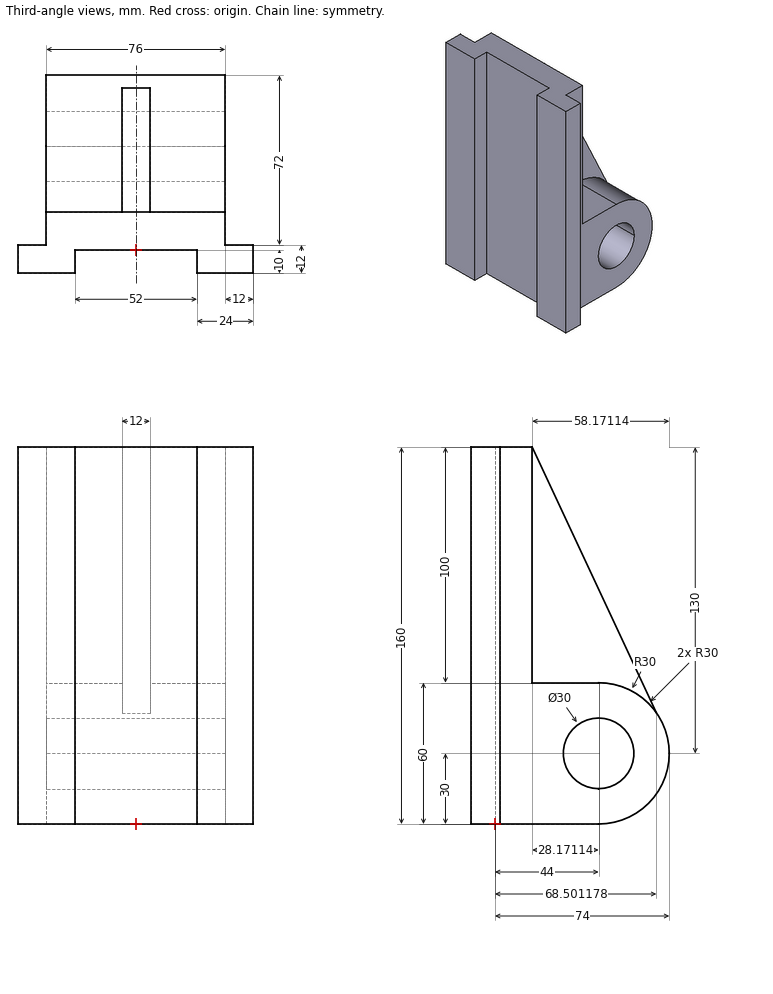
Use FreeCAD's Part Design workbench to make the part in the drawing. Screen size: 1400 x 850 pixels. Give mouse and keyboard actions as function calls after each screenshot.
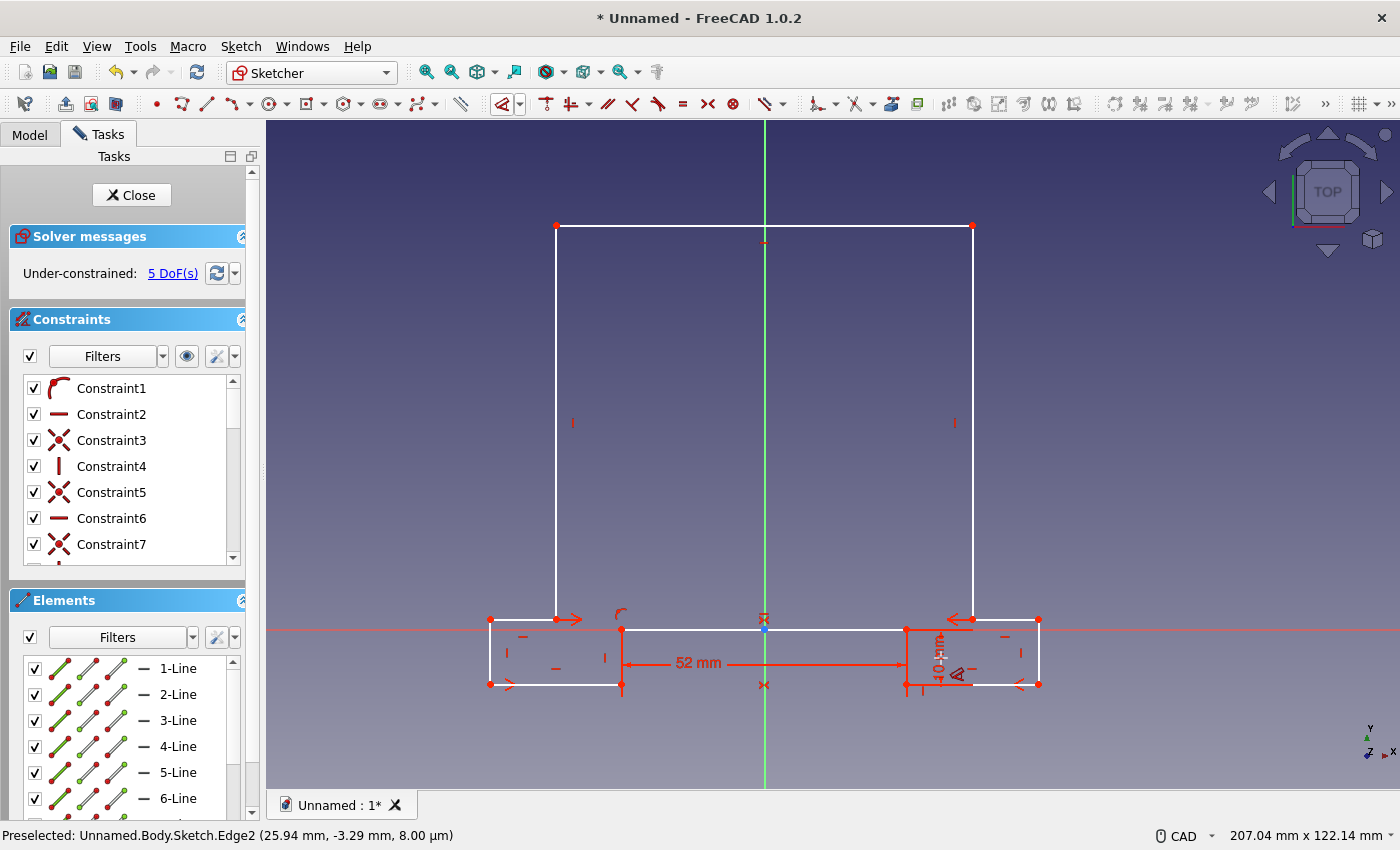
click(946, 685)
click(973, 719)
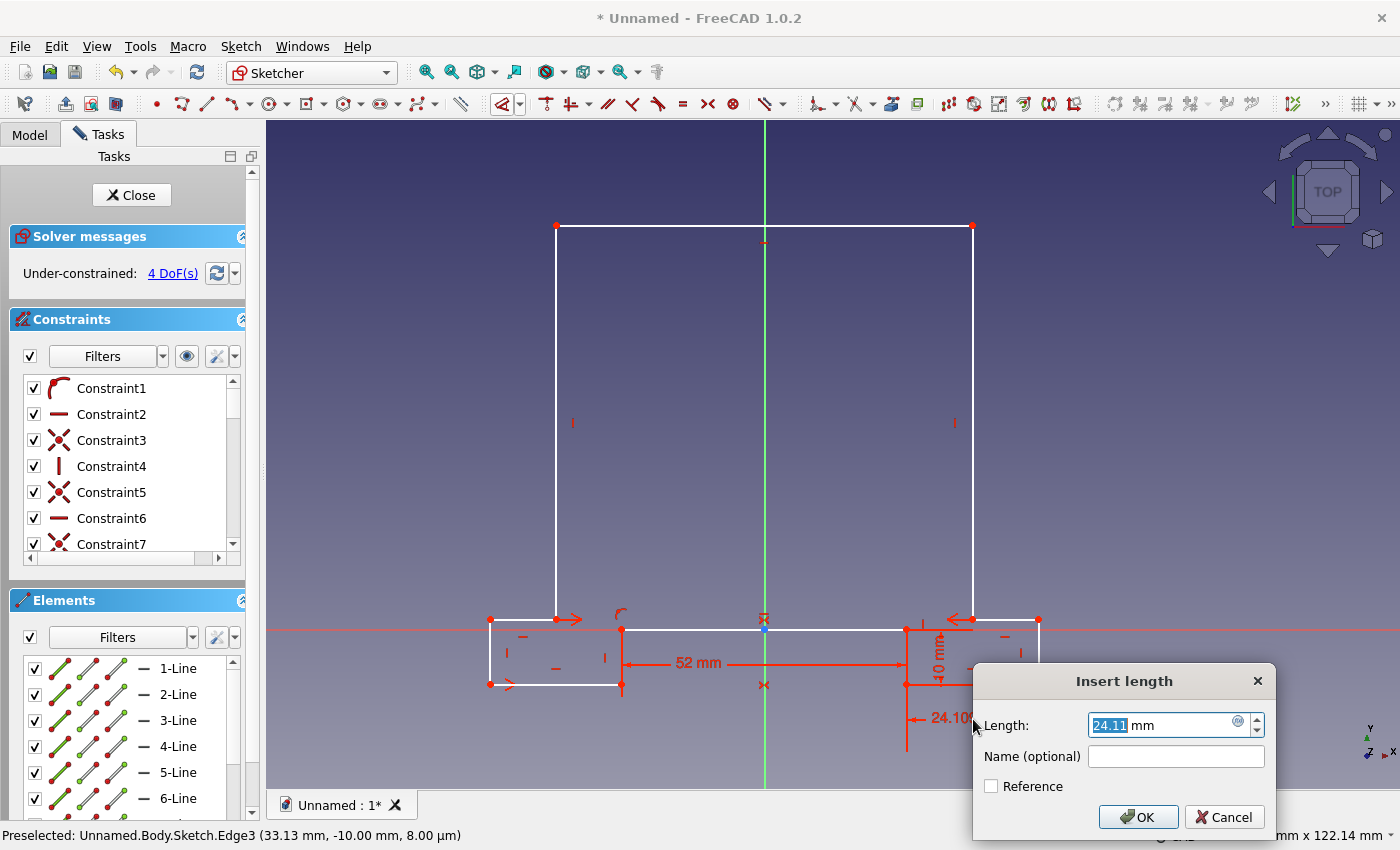
text(24)
key(Return)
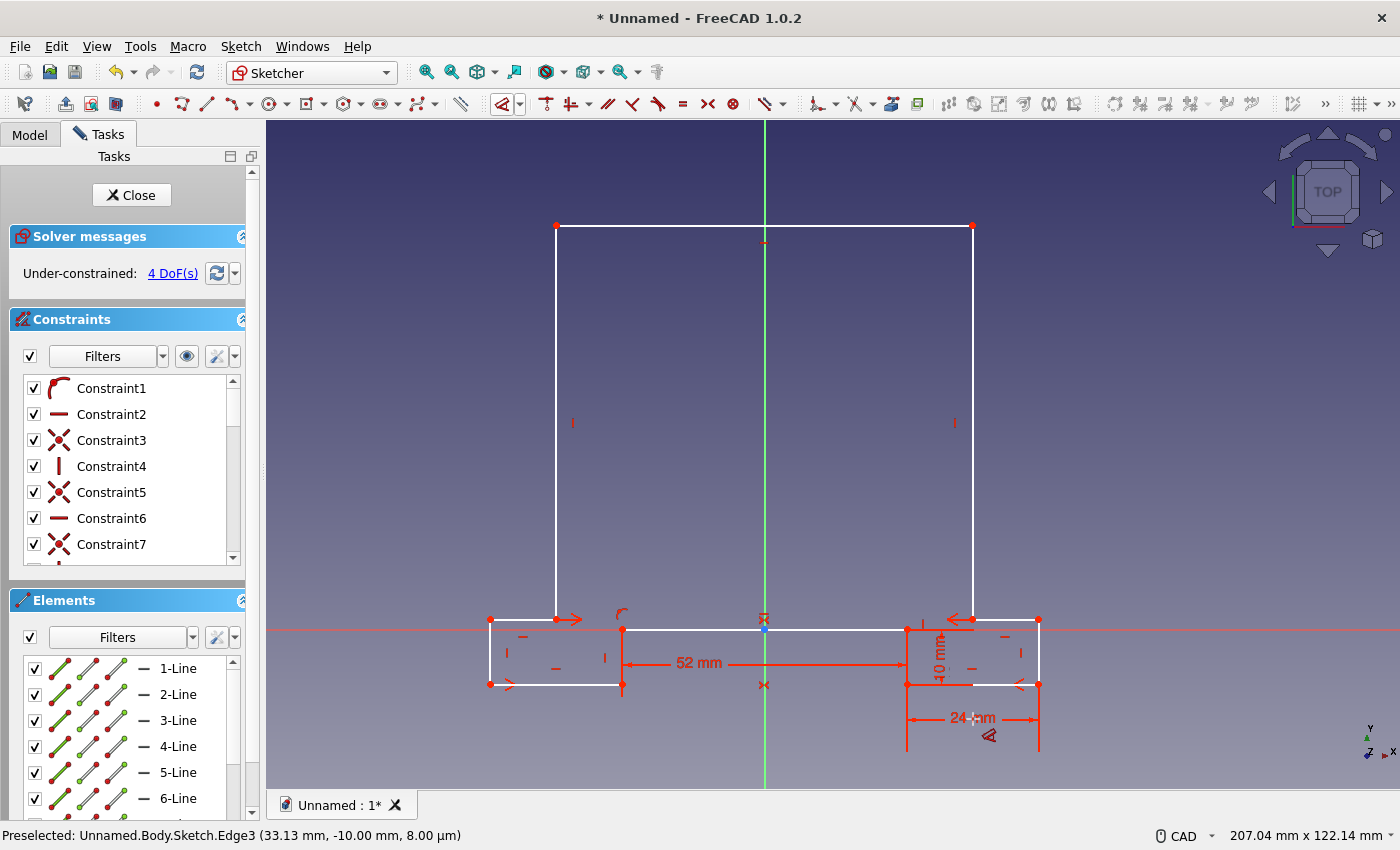
click(1039, 665)
click(1073, 652)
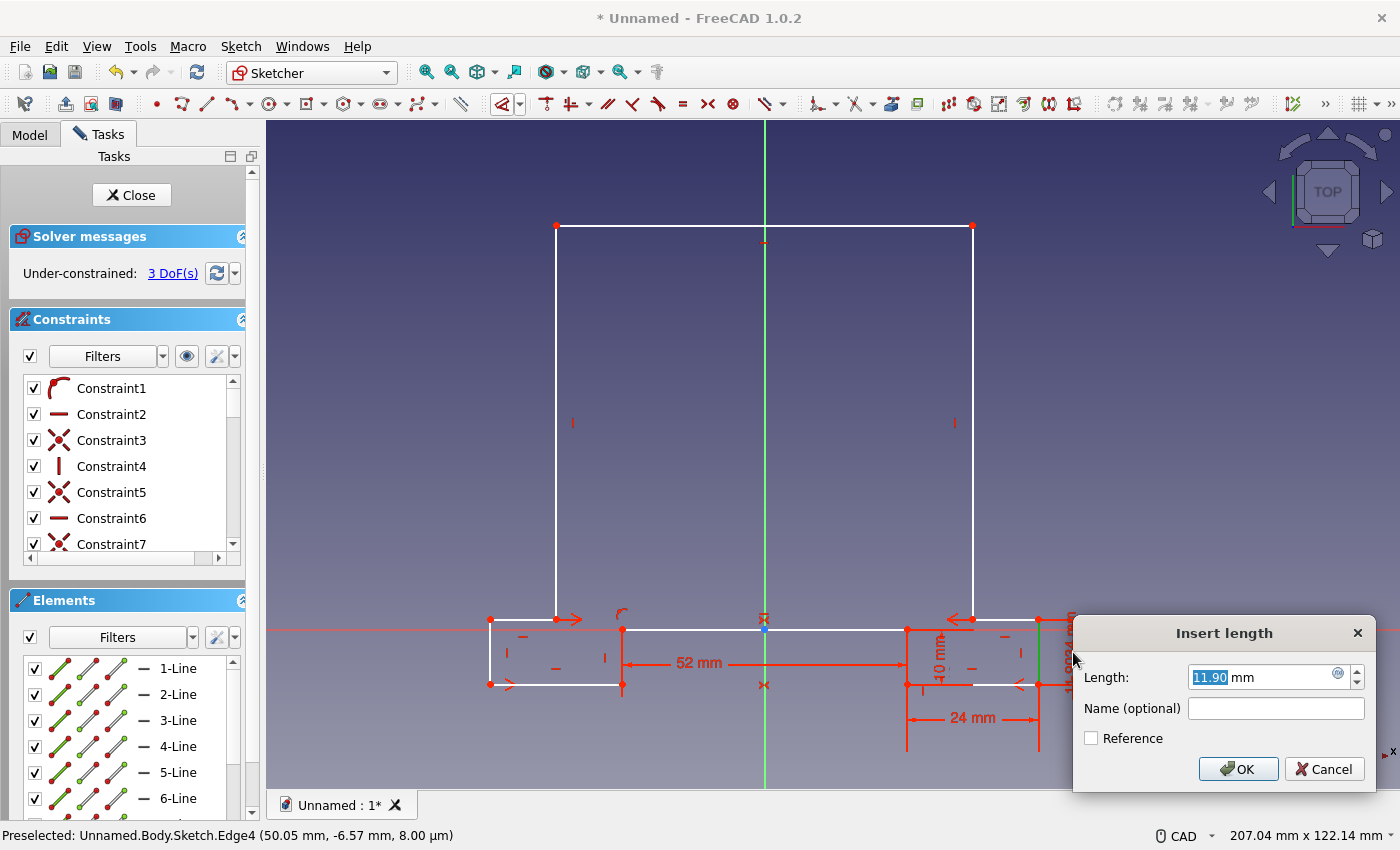
text(12)
key(Return)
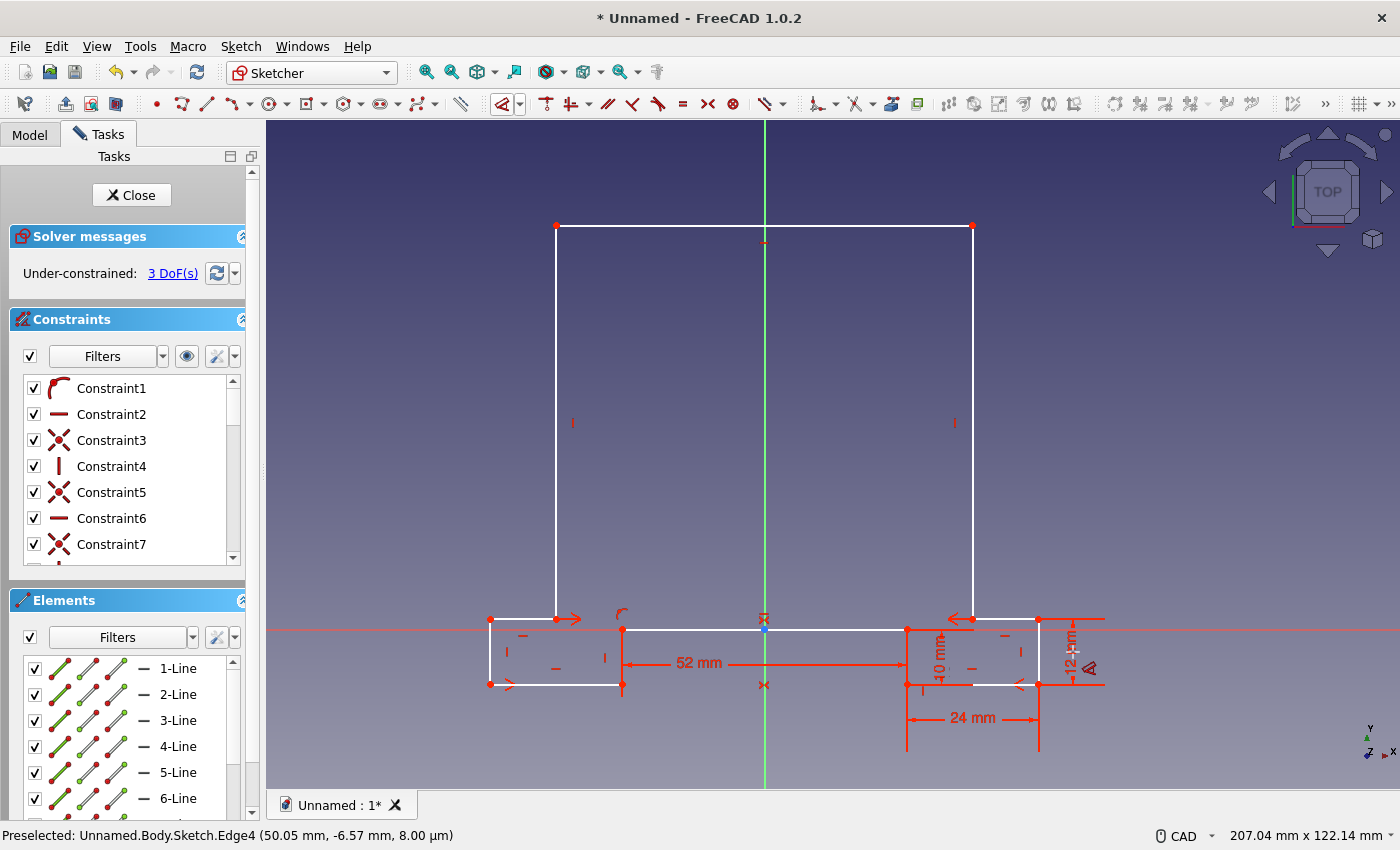
scroll(1019, 619, up, 2)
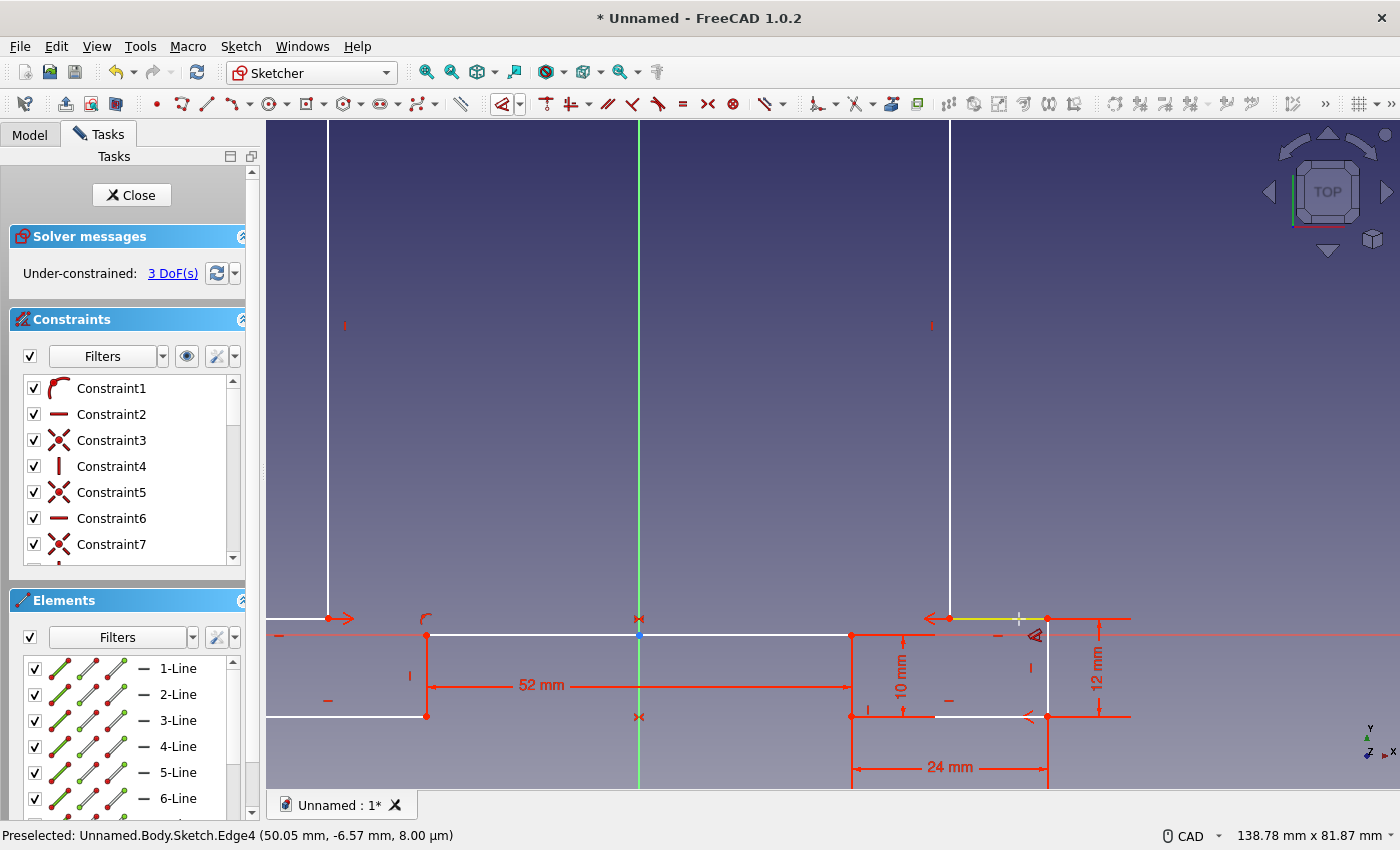
click(1018, 619)
click(999, 653)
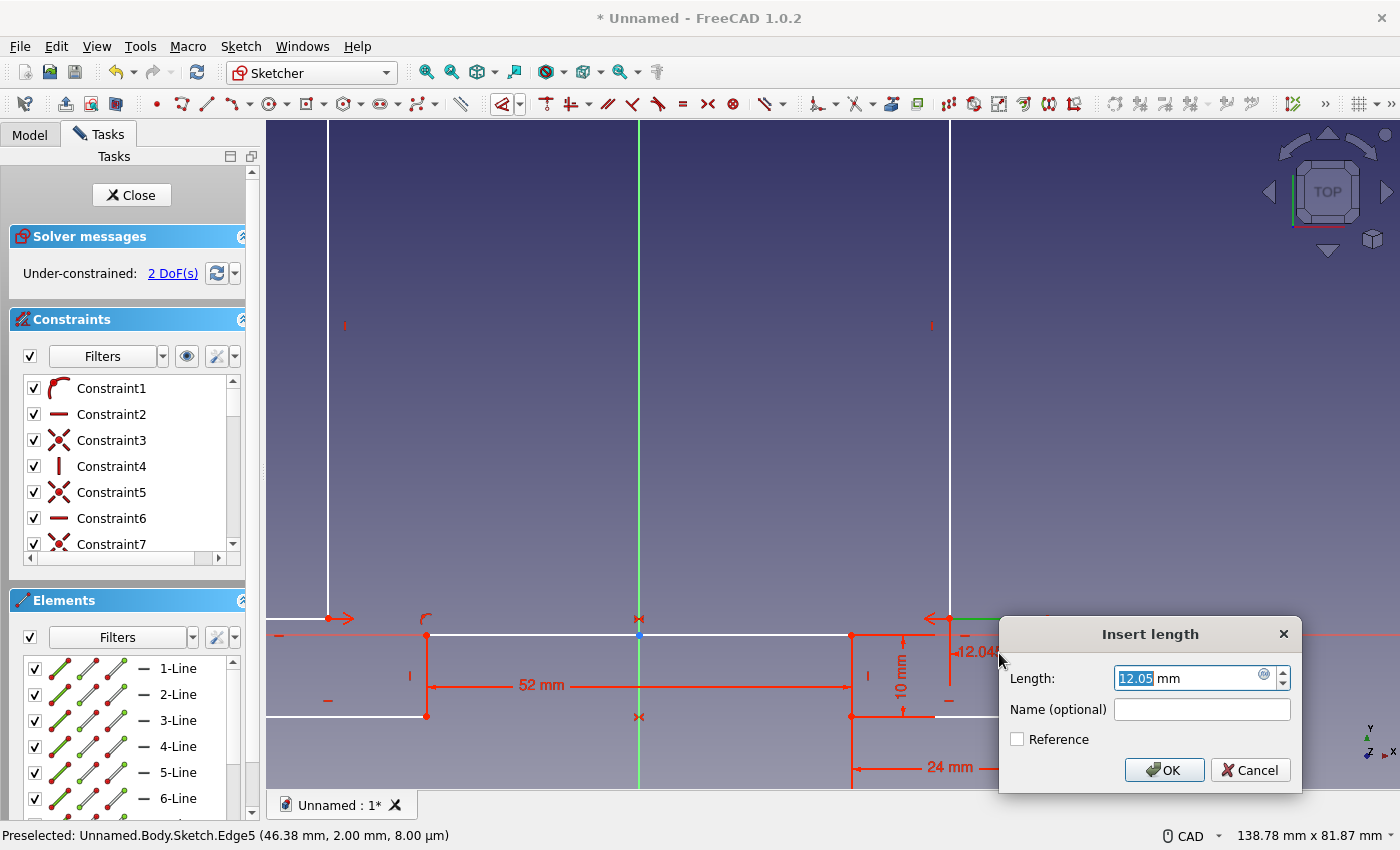
text(12)
key(Return)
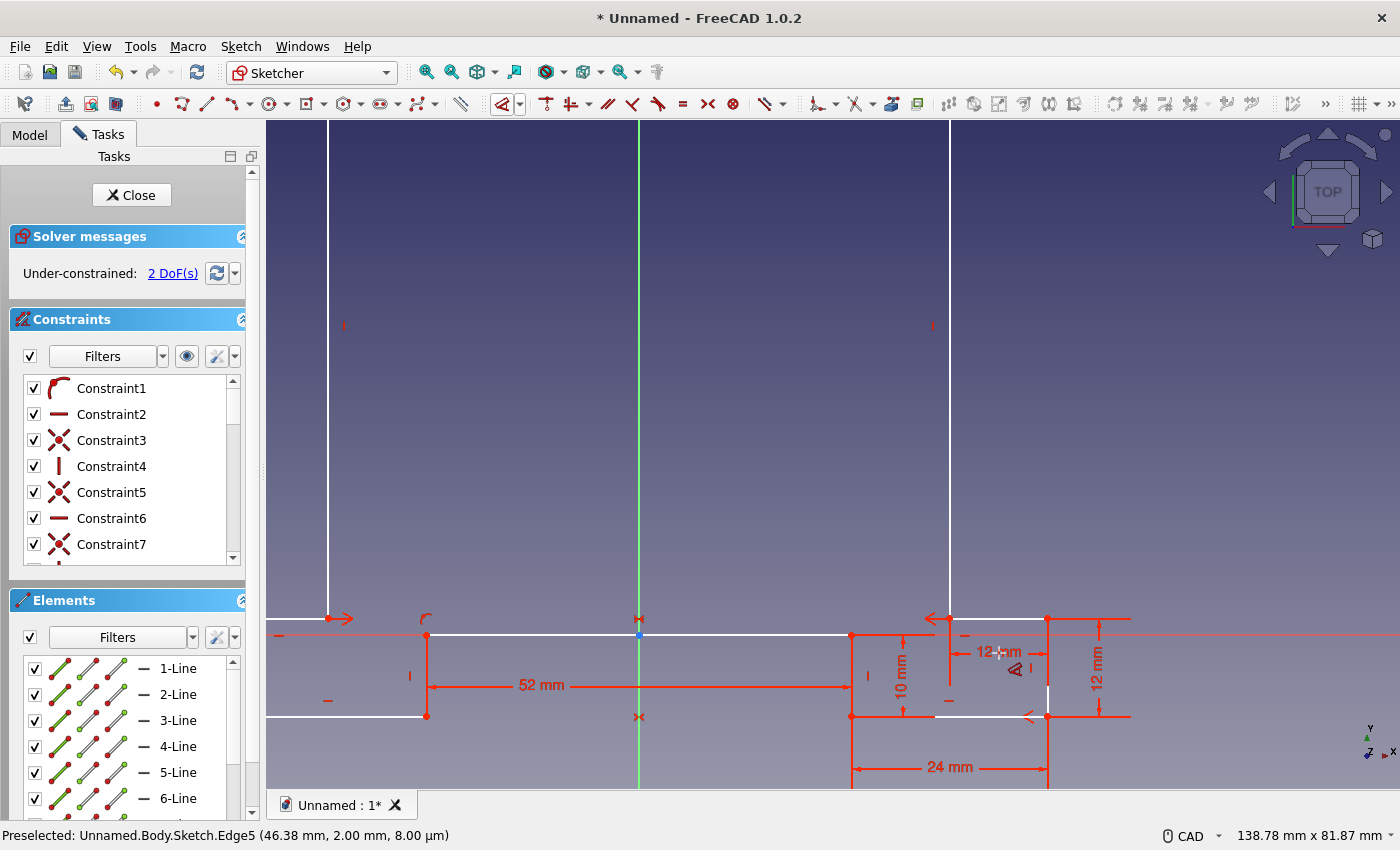
click(950, 443)
click(984, 383)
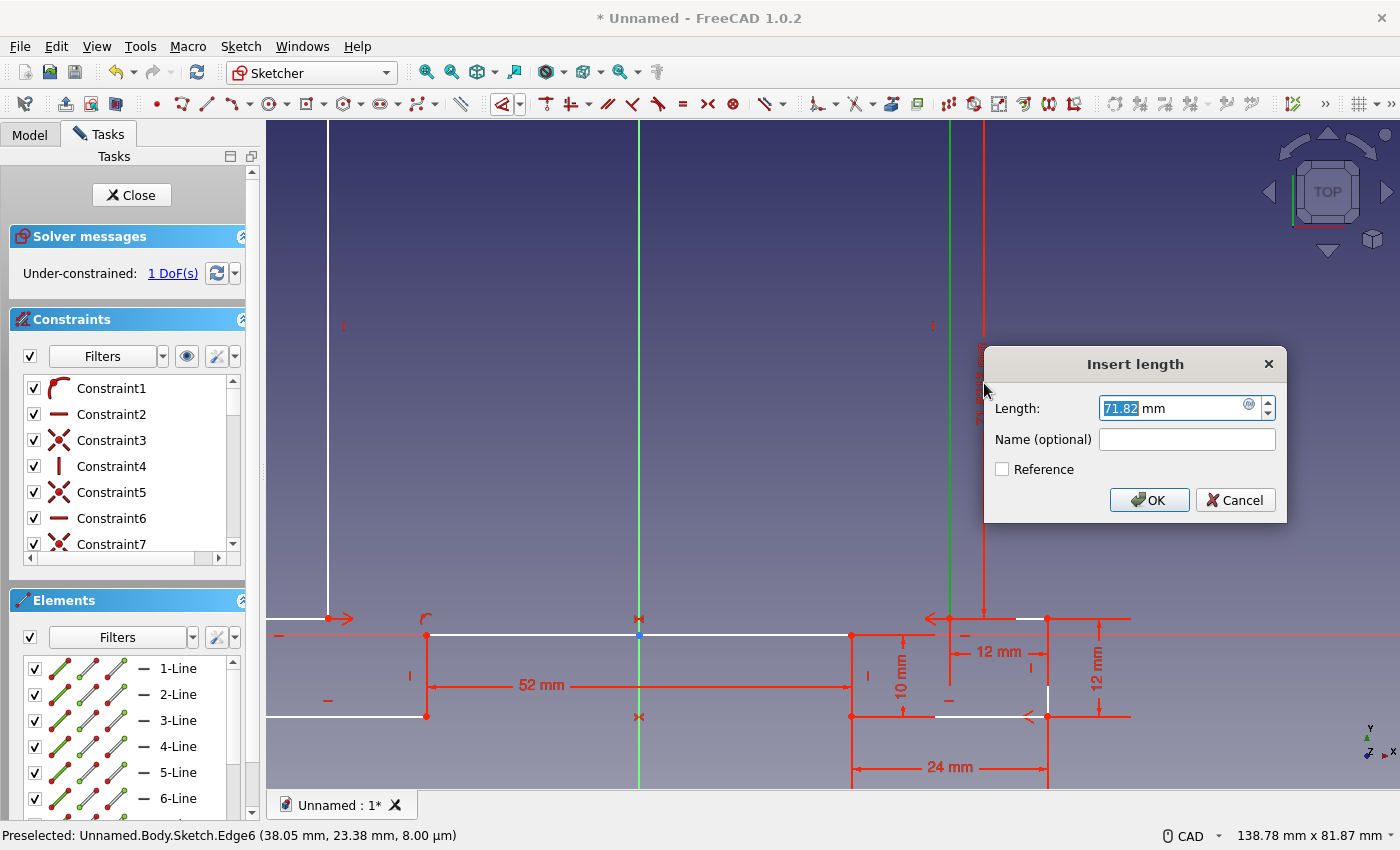
text(72)
key(Return)